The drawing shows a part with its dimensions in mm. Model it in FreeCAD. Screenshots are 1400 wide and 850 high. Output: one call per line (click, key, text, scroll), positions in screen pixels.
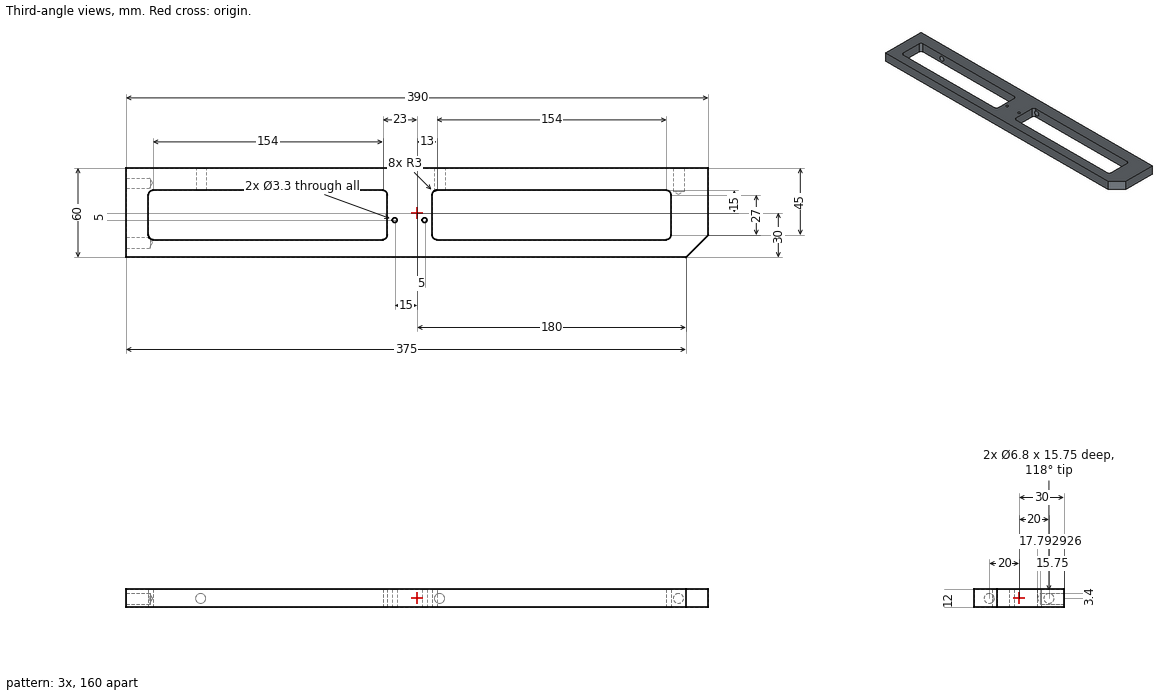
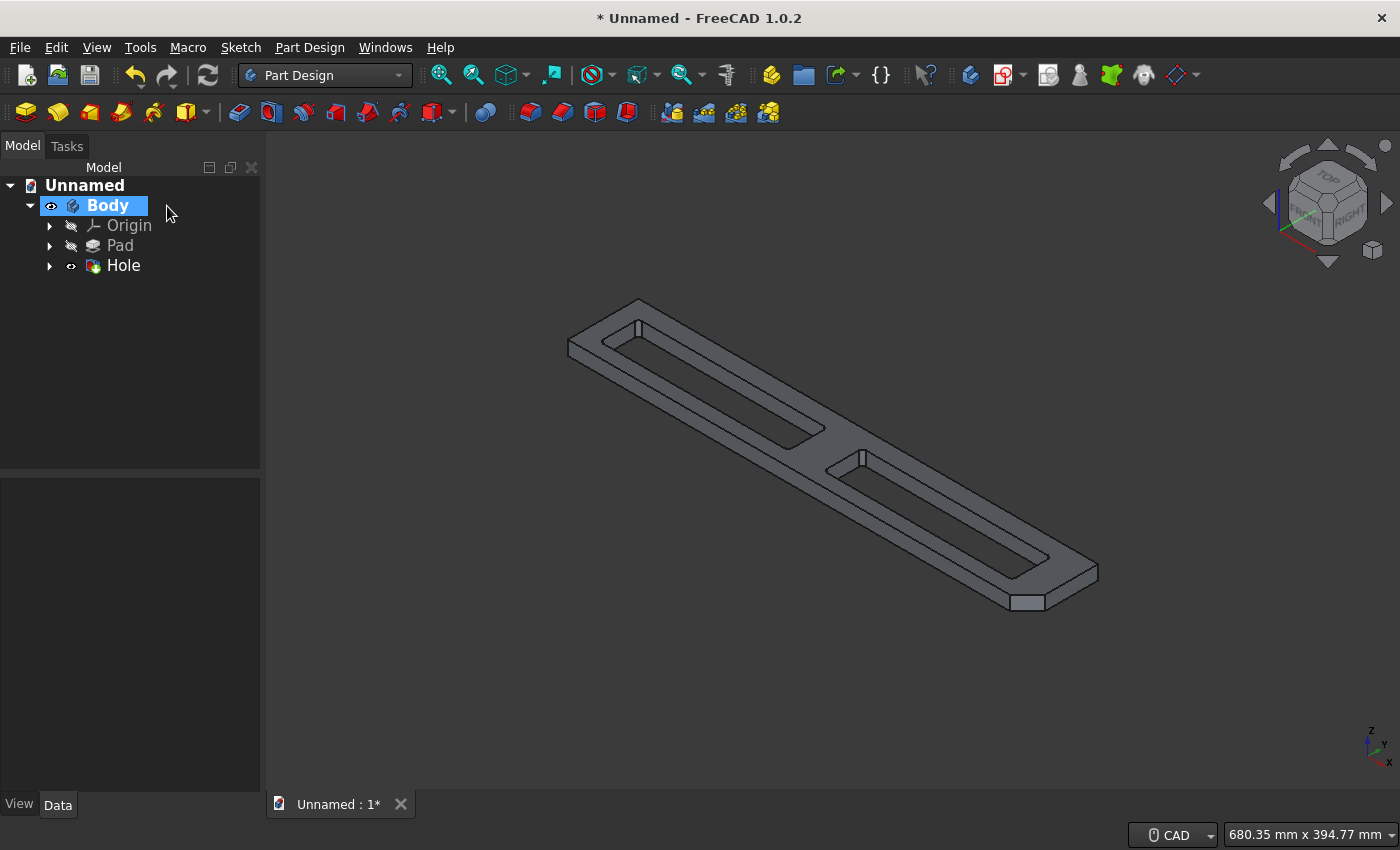
click(853, 439)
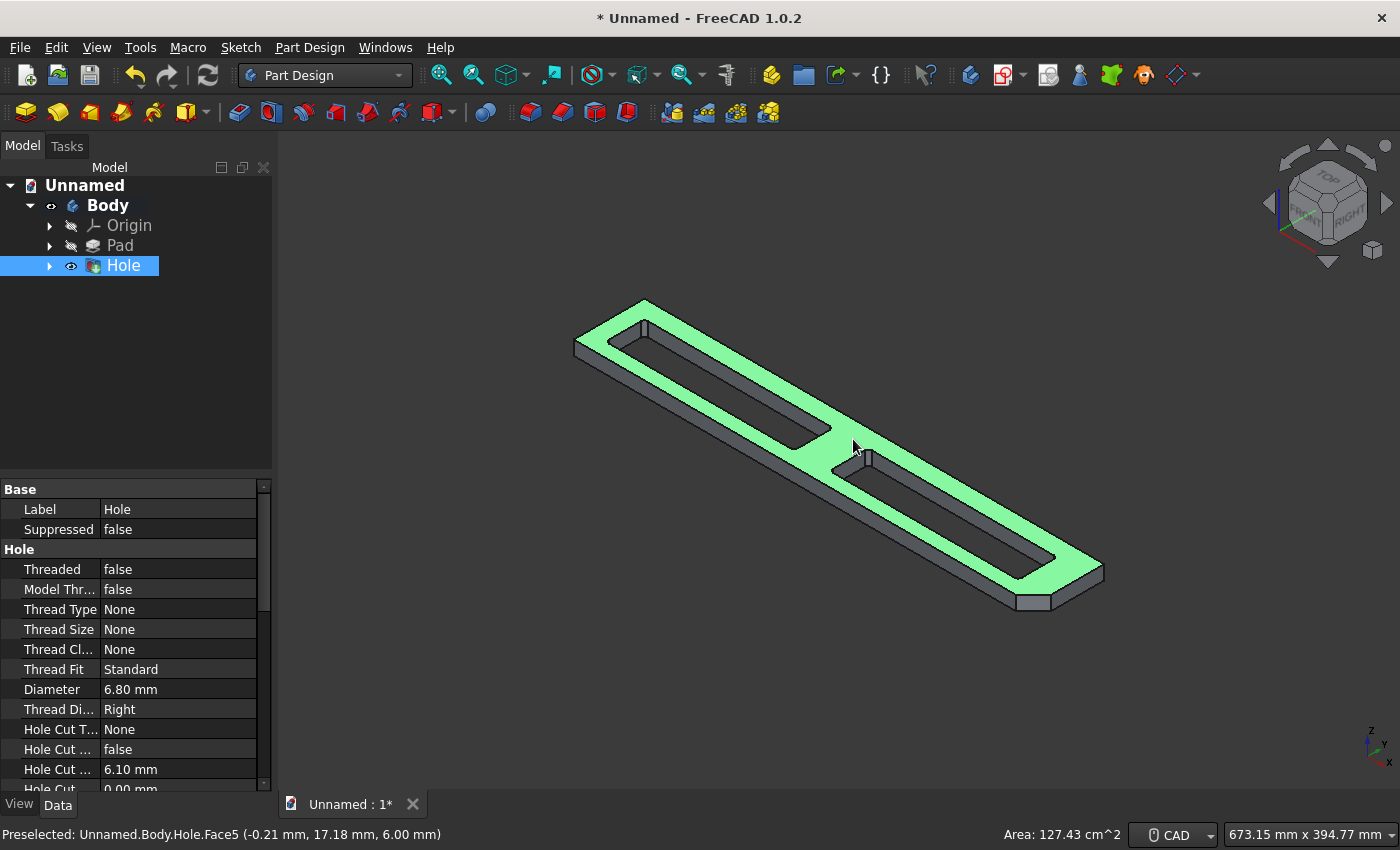
click(1004, 76)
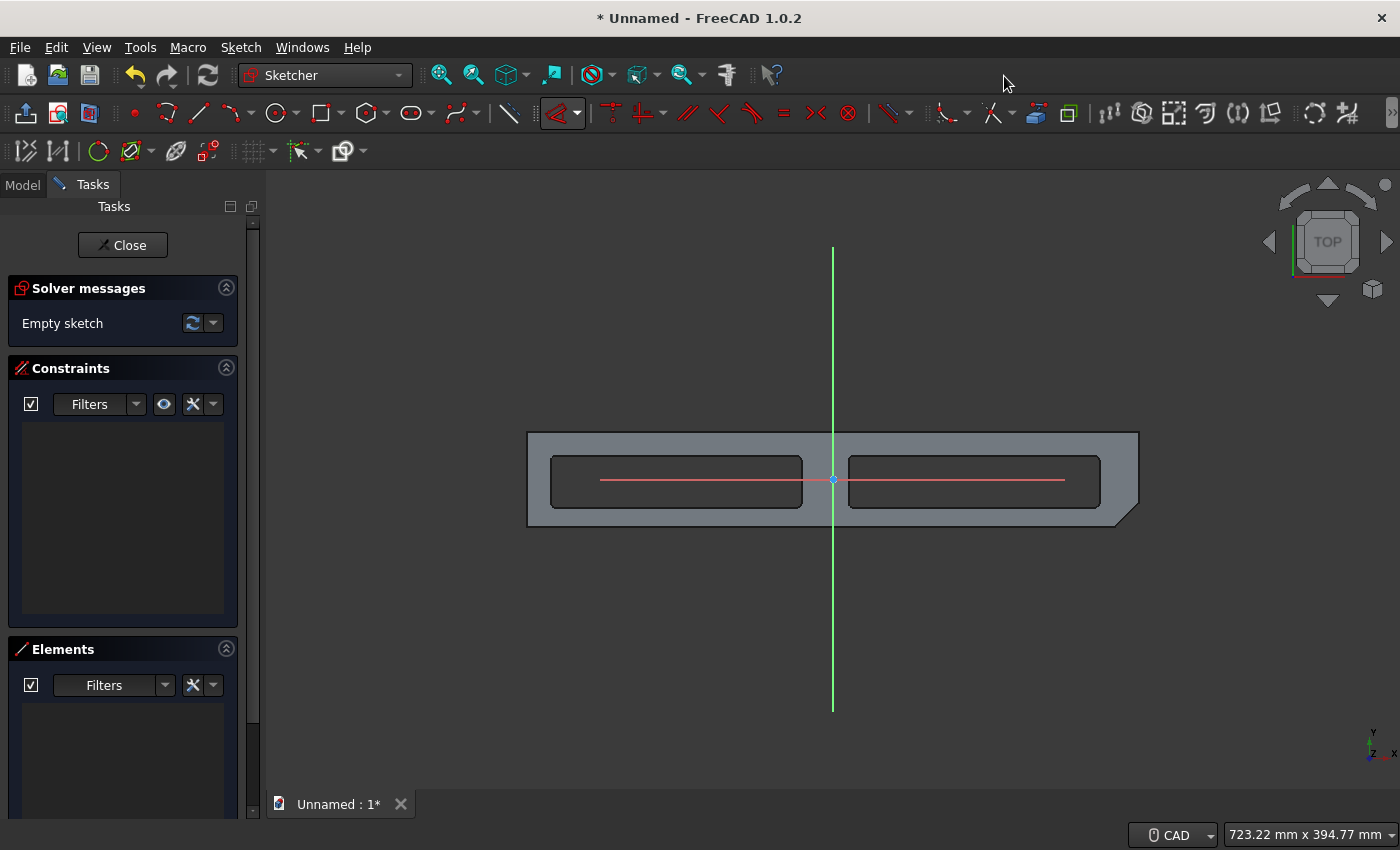
scroll(828, 485, up, 15)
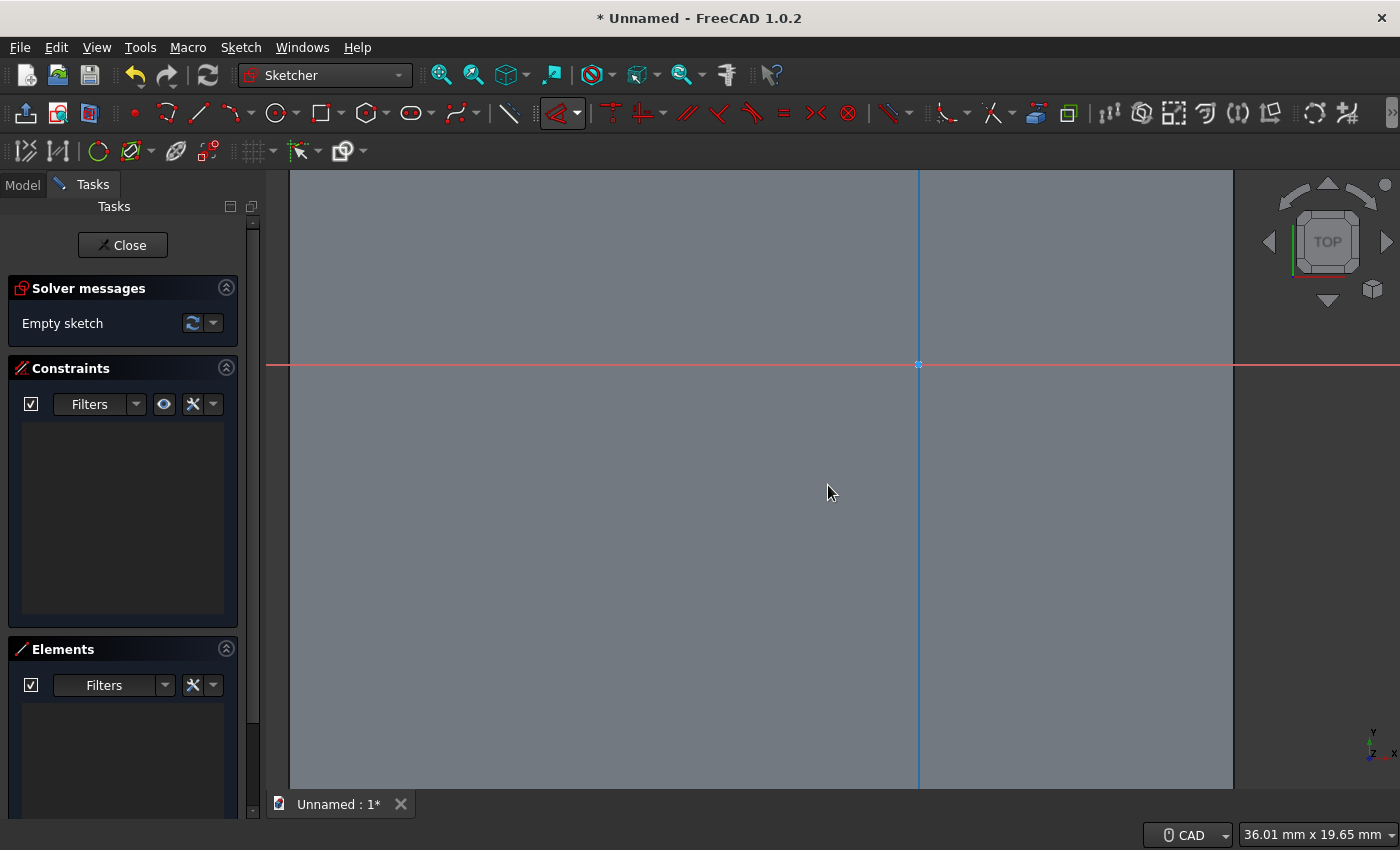
click(276, 114)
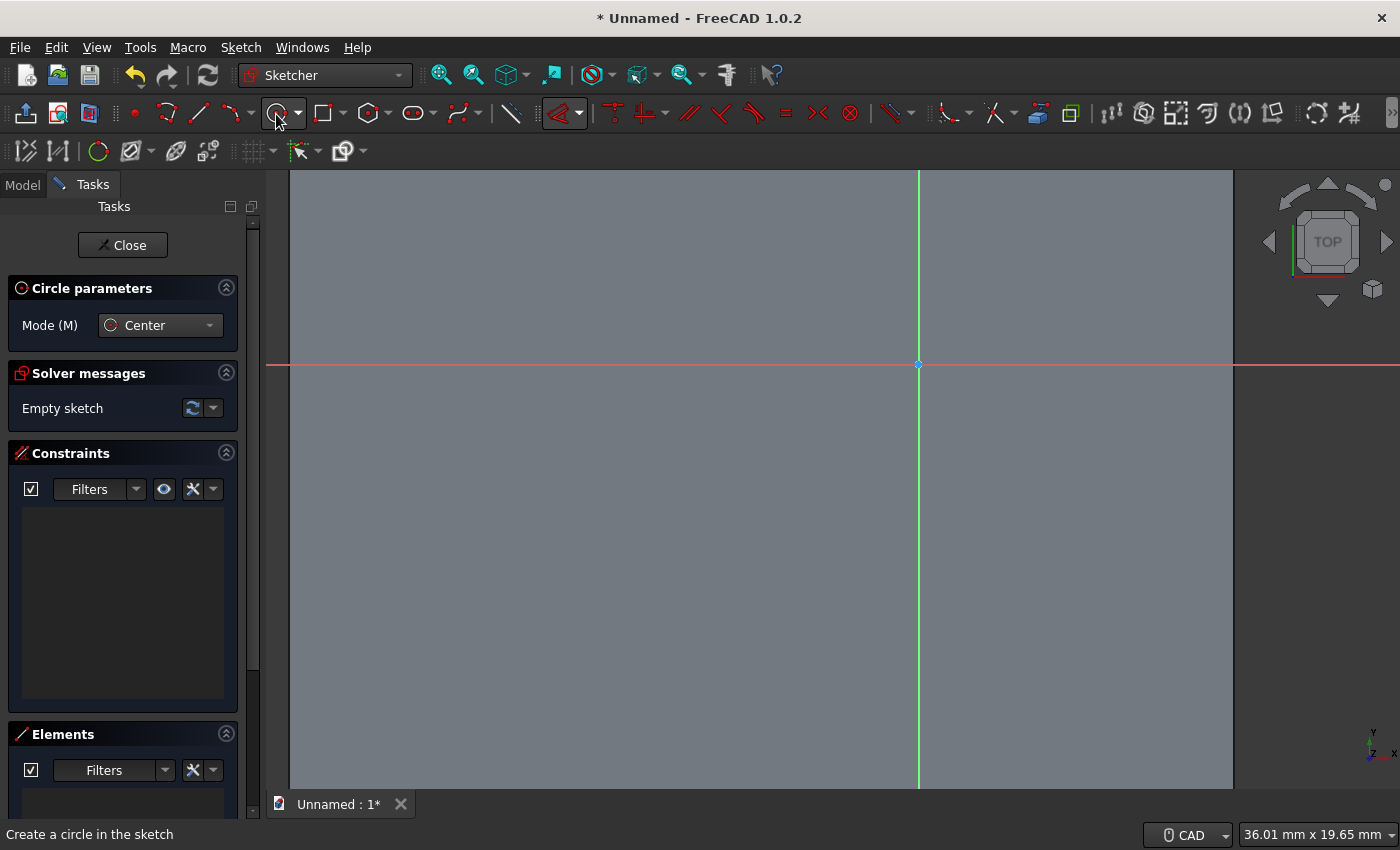
click(447, 522)
move(483, 486)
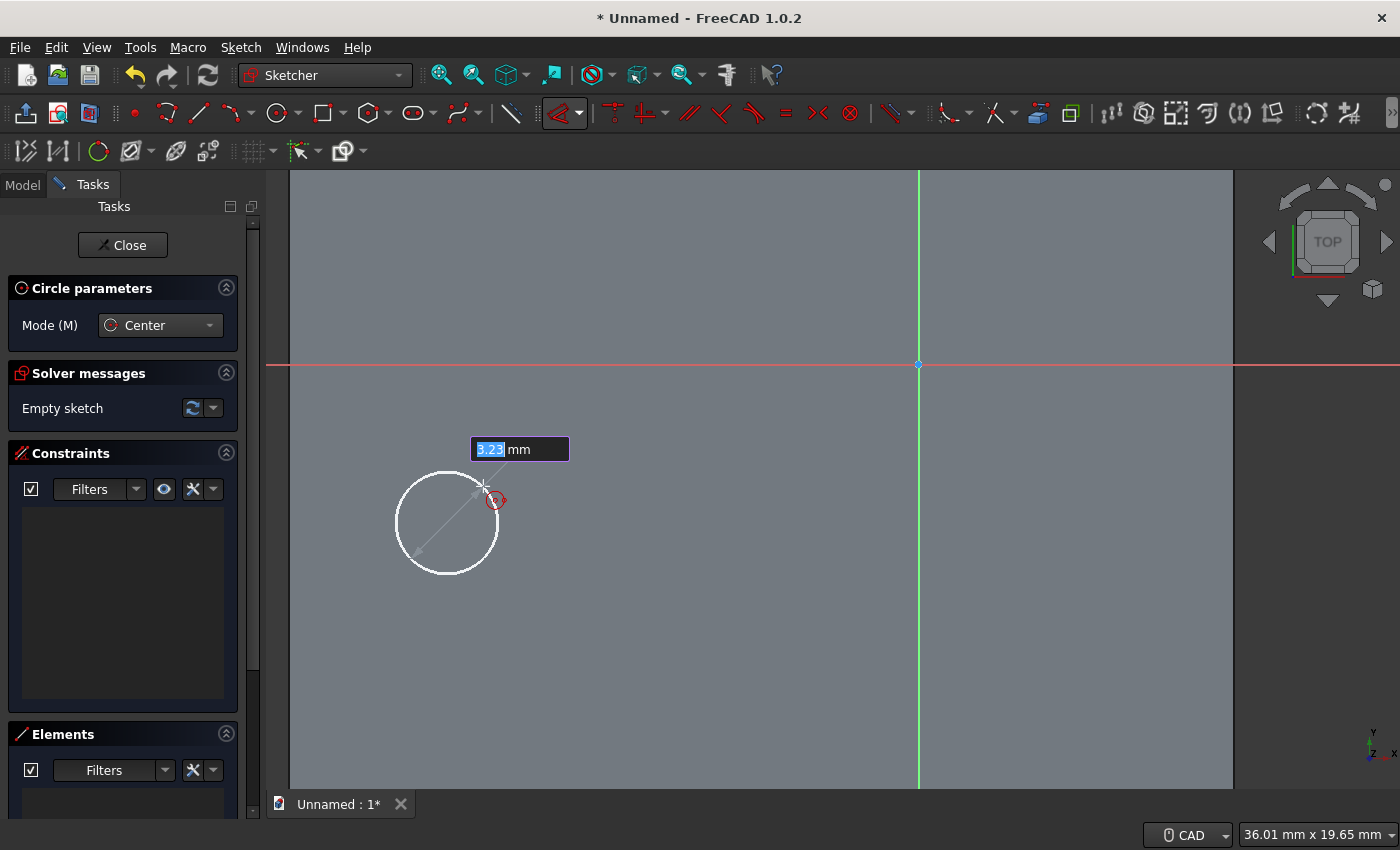
text(3.3)
key(Return)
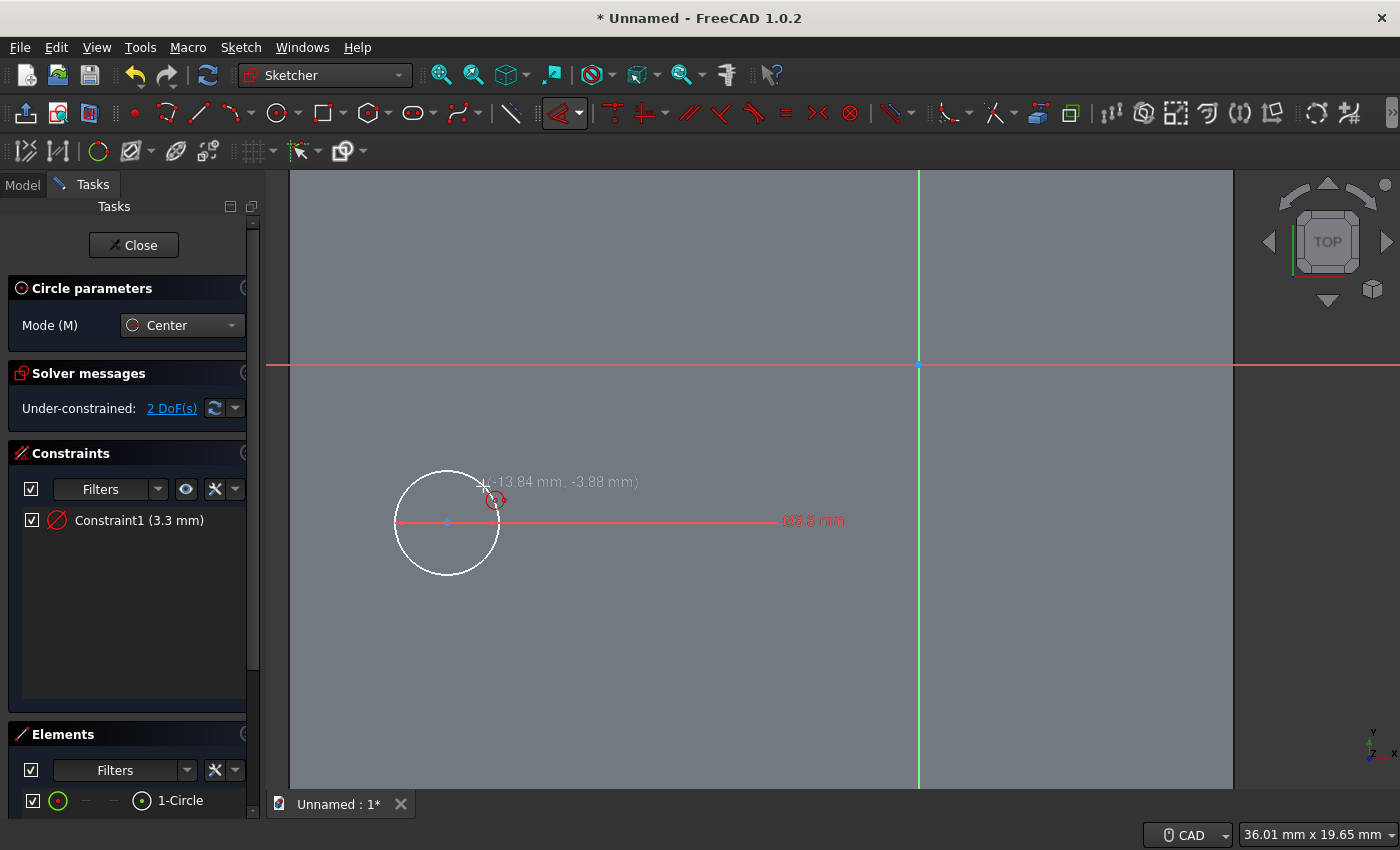
click(1076, 522)
move(1113, 486)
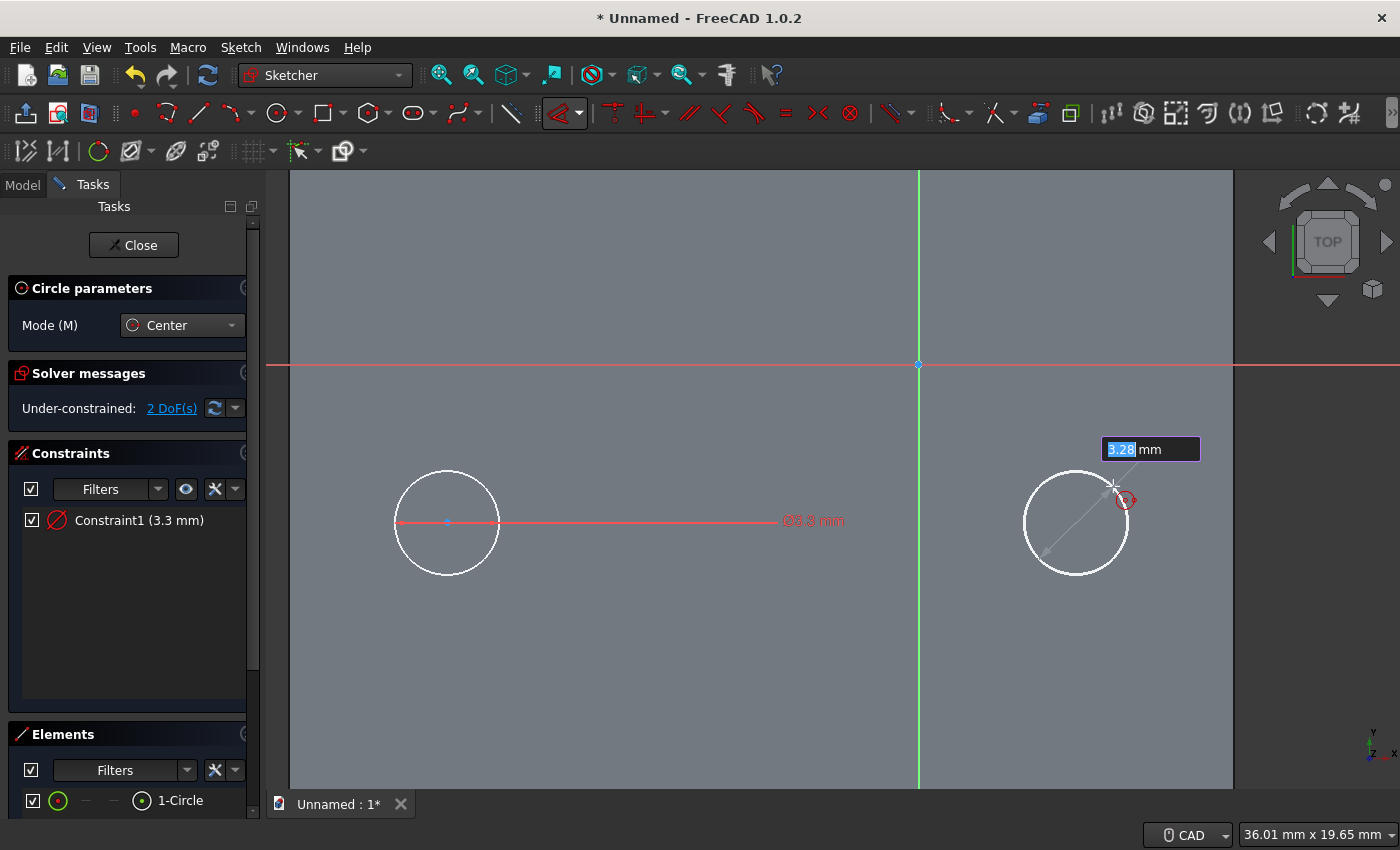
text(3.3)
key(Return)
key(Escape)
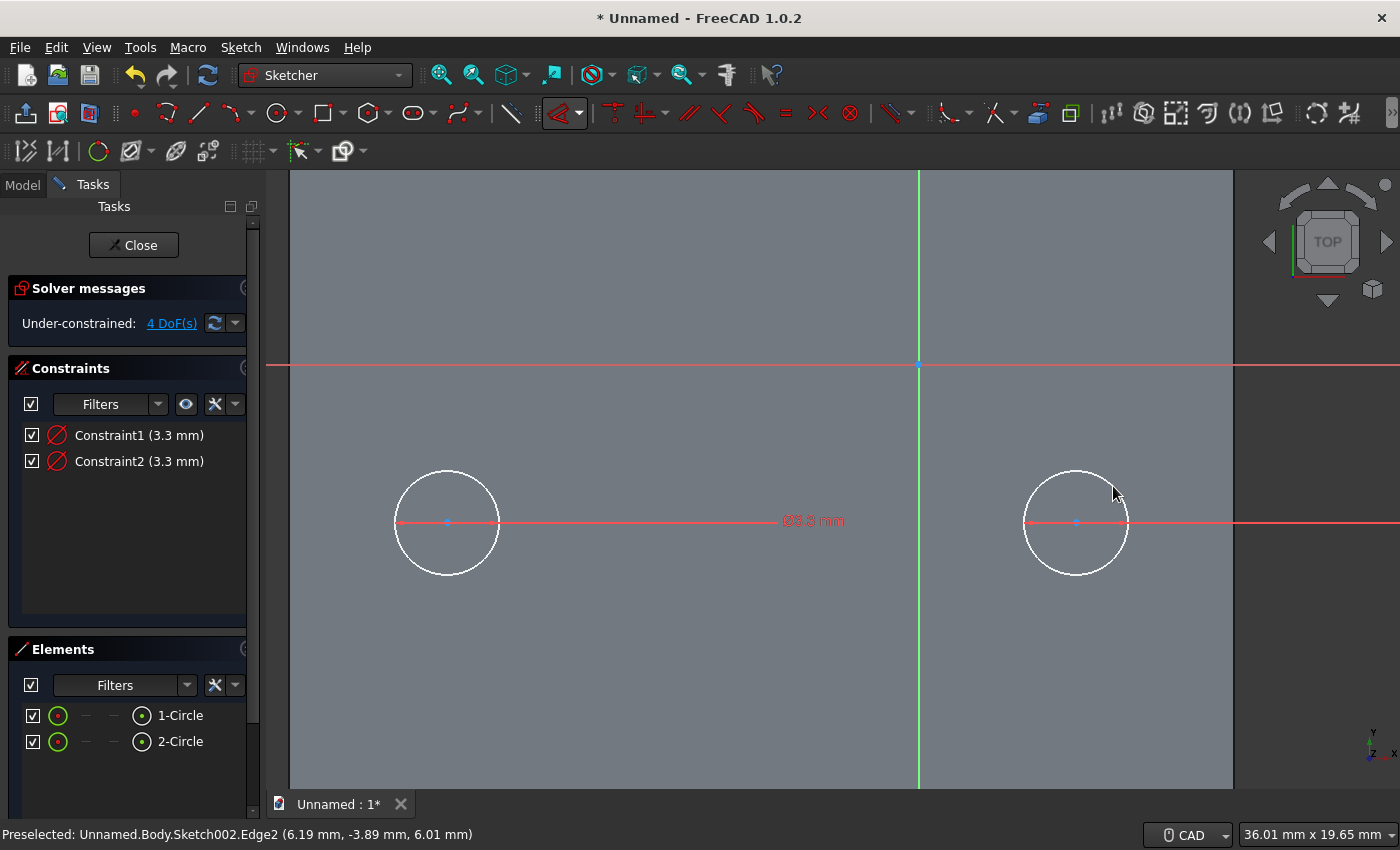
click(447, 523)